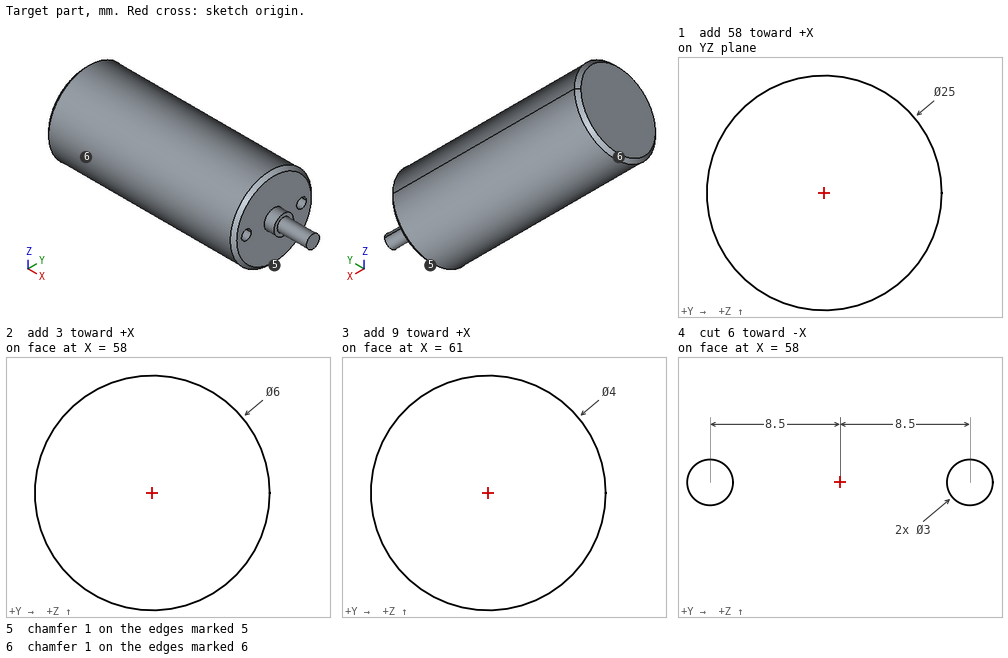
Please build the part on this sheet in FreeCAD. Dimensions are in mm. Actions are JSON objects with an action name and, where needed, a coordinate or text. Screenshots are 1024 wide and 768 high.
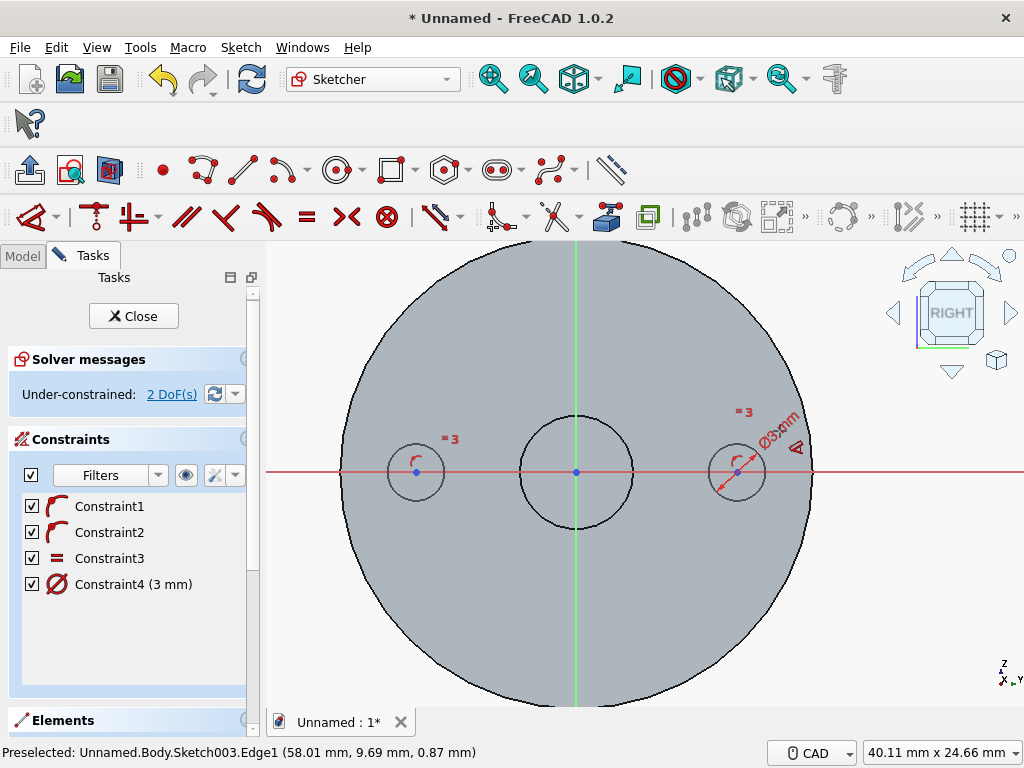
{"action": "left_click", "coordinate": [737, 472]}
{"action": "left_click", "coordinate": [657, 506]}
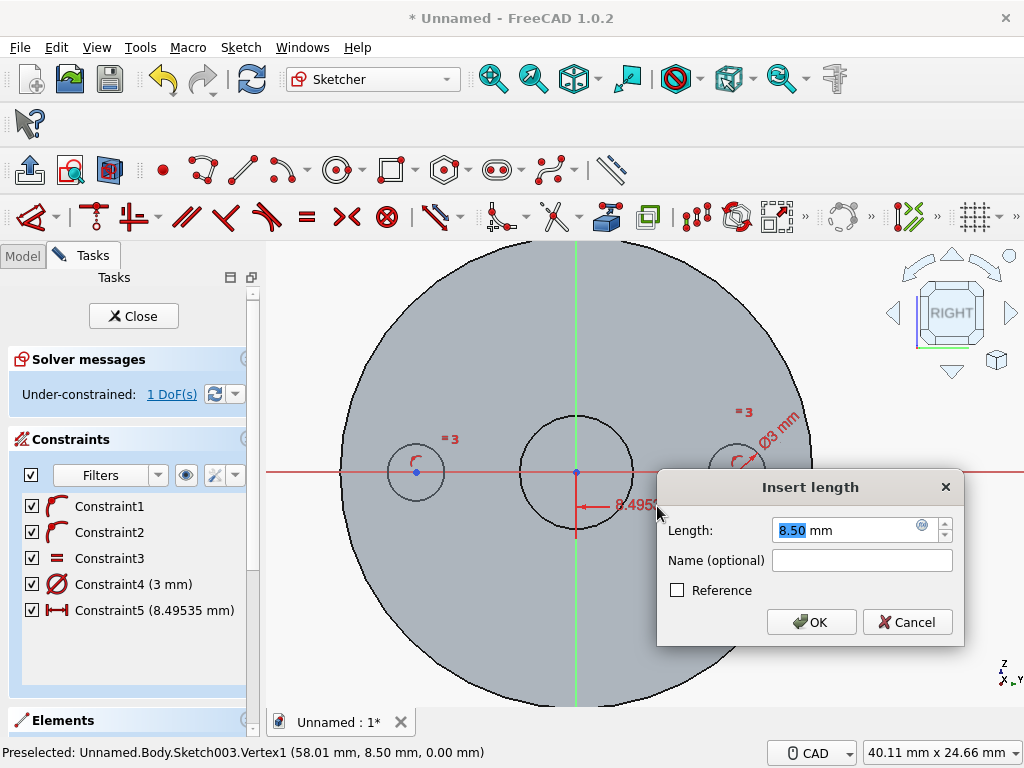
{"action": "type", "text": "8.5"}
{"action": "key", "text": "Return"}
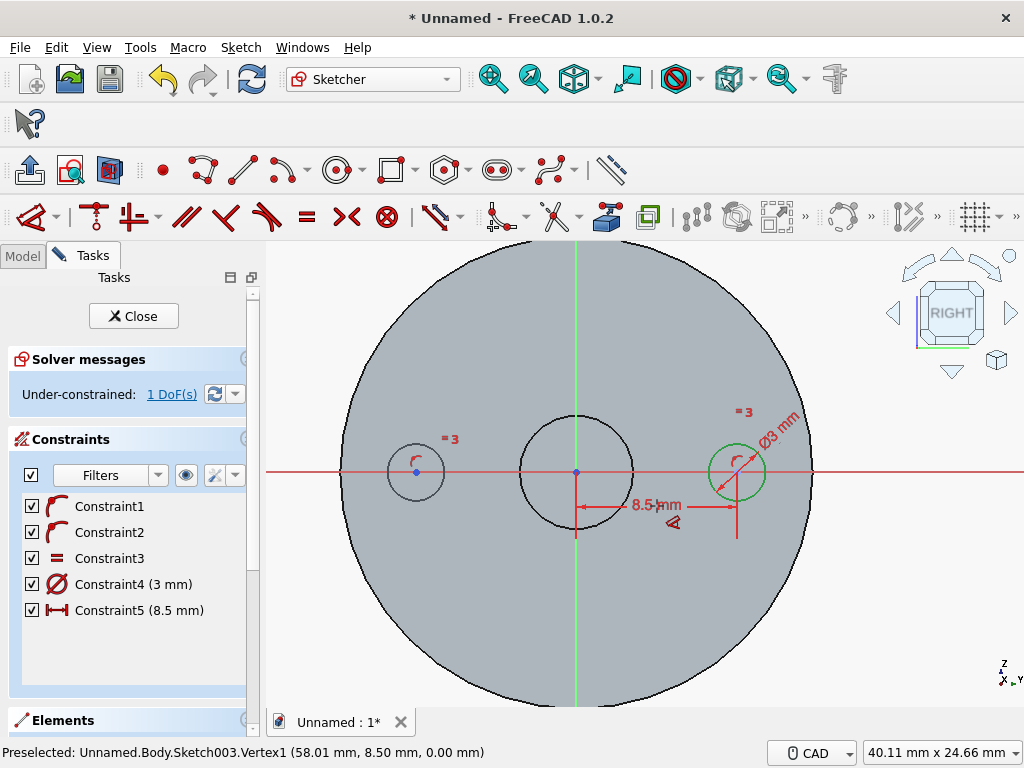
{"action": "left_click", "coordinate": [416, 472]}
{"action": "left_click", "coordinate": [496, 506]}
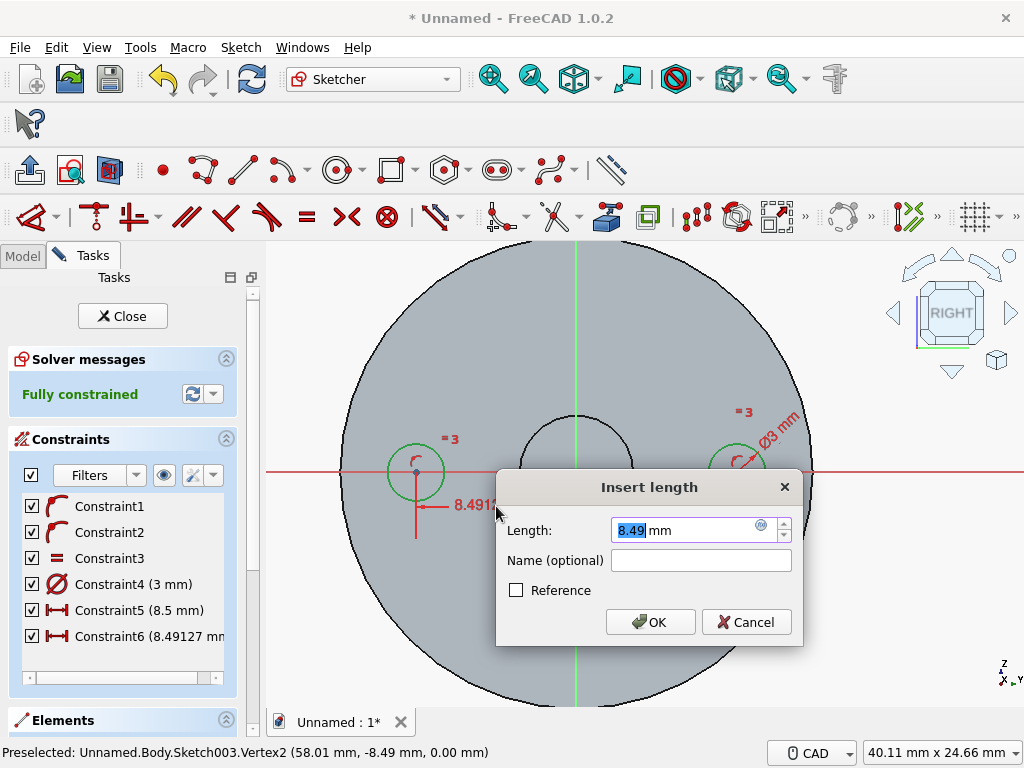
{"action": "type", "text": "8.5"}
{"action": "key", "text": "Return"}
{"action": "key", "text": "Escape"}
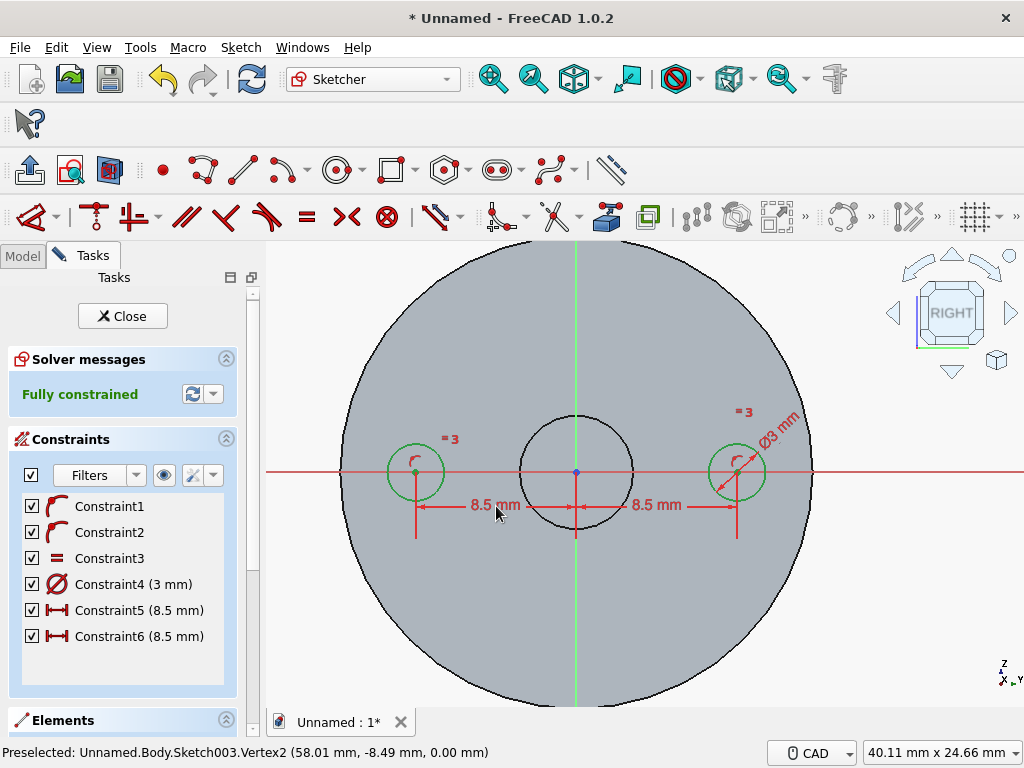
{"action": "left_click", "coordinate": [123, 316]}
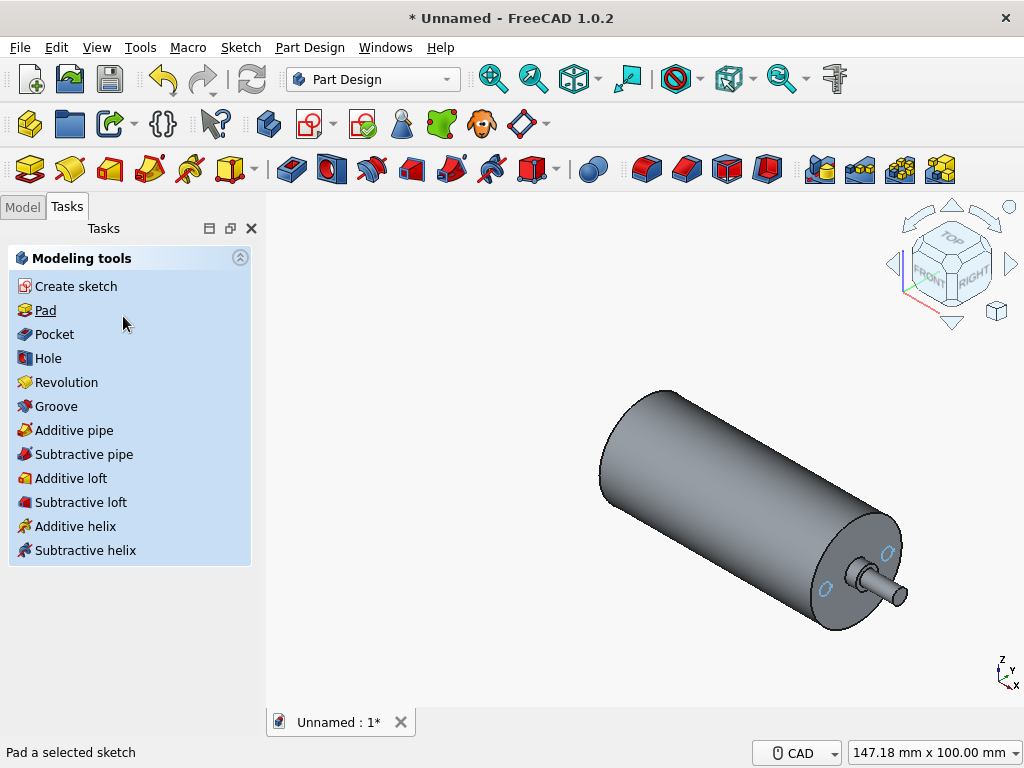
{"action": "left_click", "coordinate": [292, 170]}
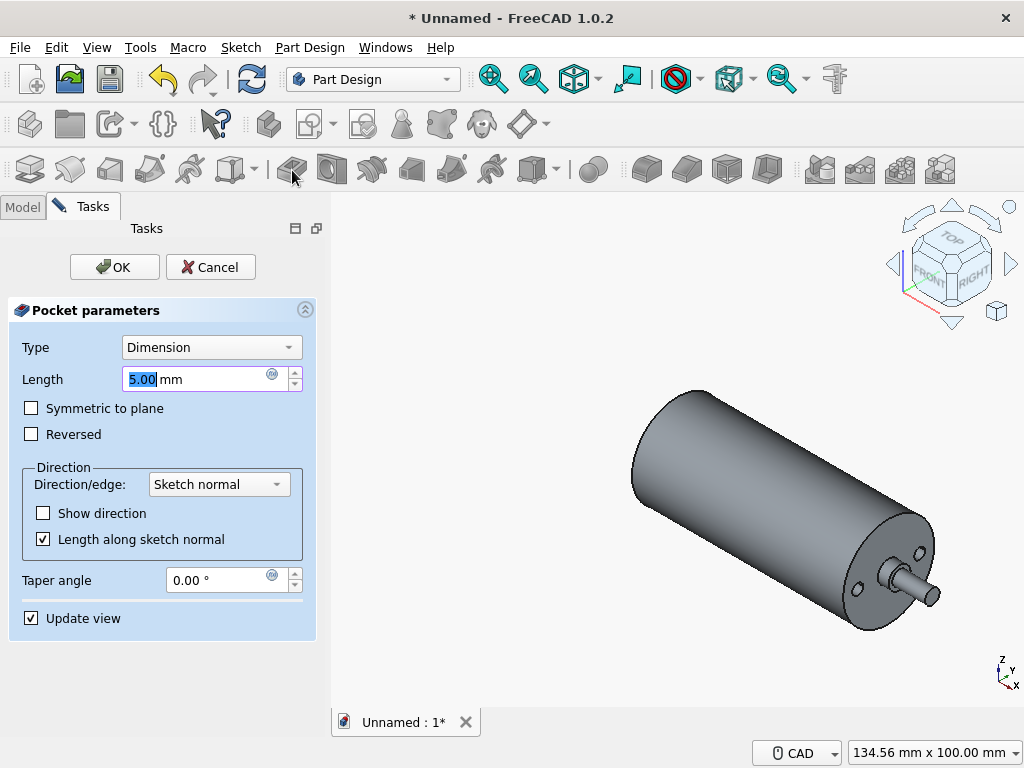
{"action": "type", "text": "6"}
{"action": "key", "text": "Tab"}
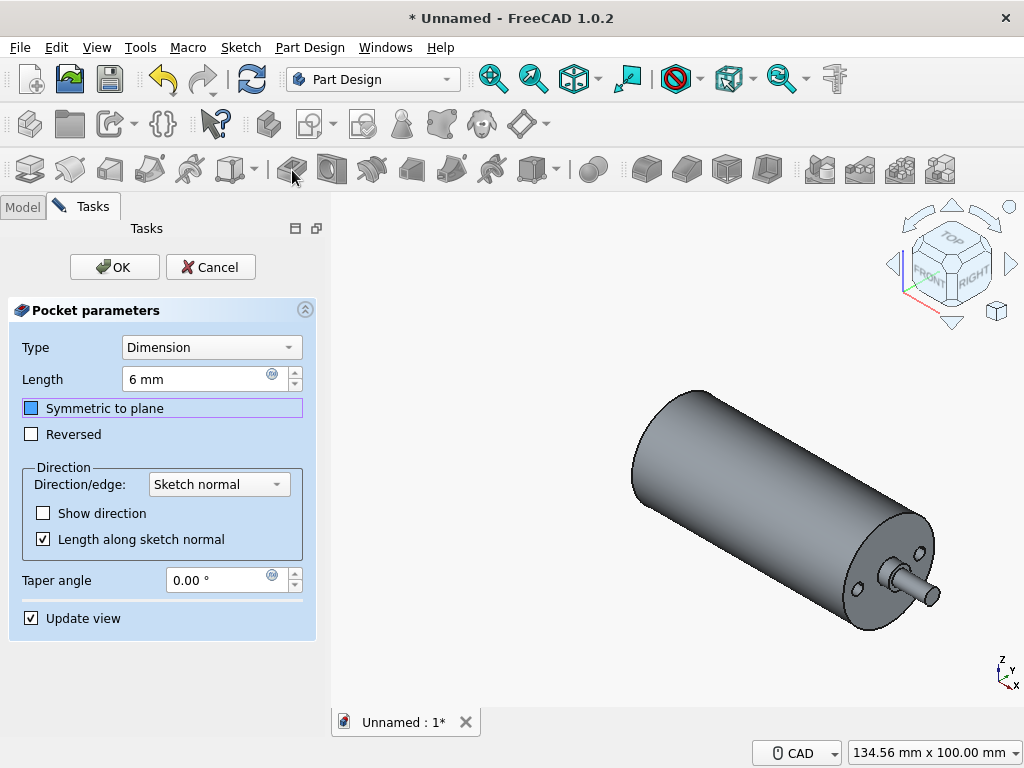
{"action": "left_click", "coordinate": [115, 267]}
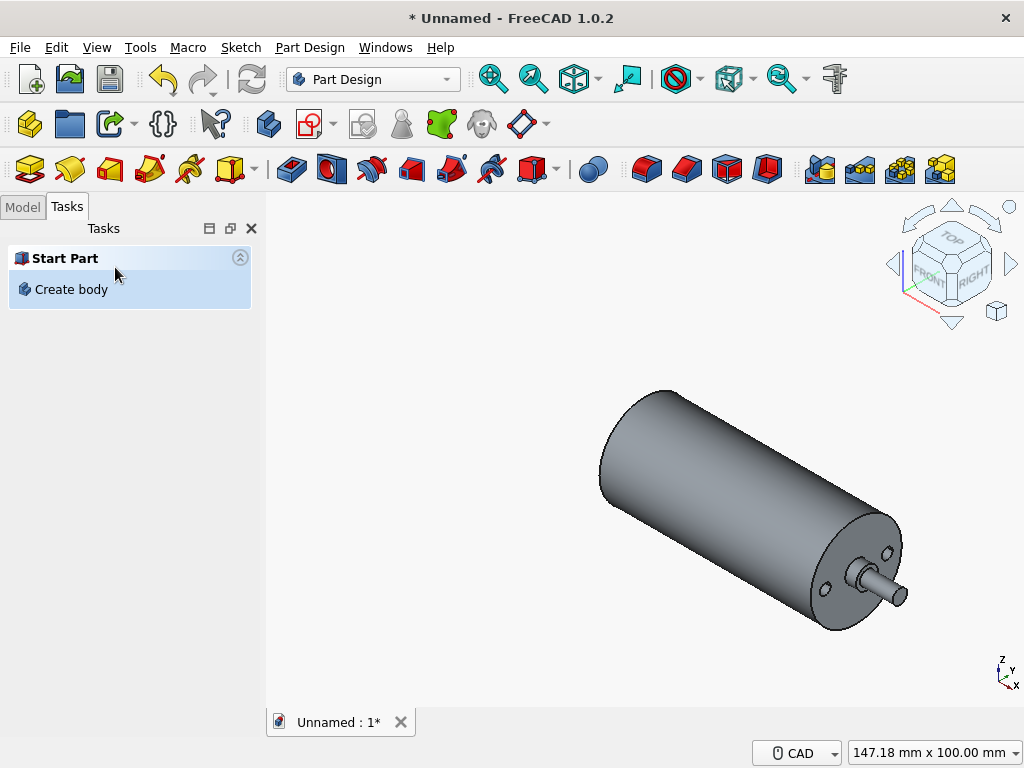
{"action": "left_click", "coordinate": [811, 597]}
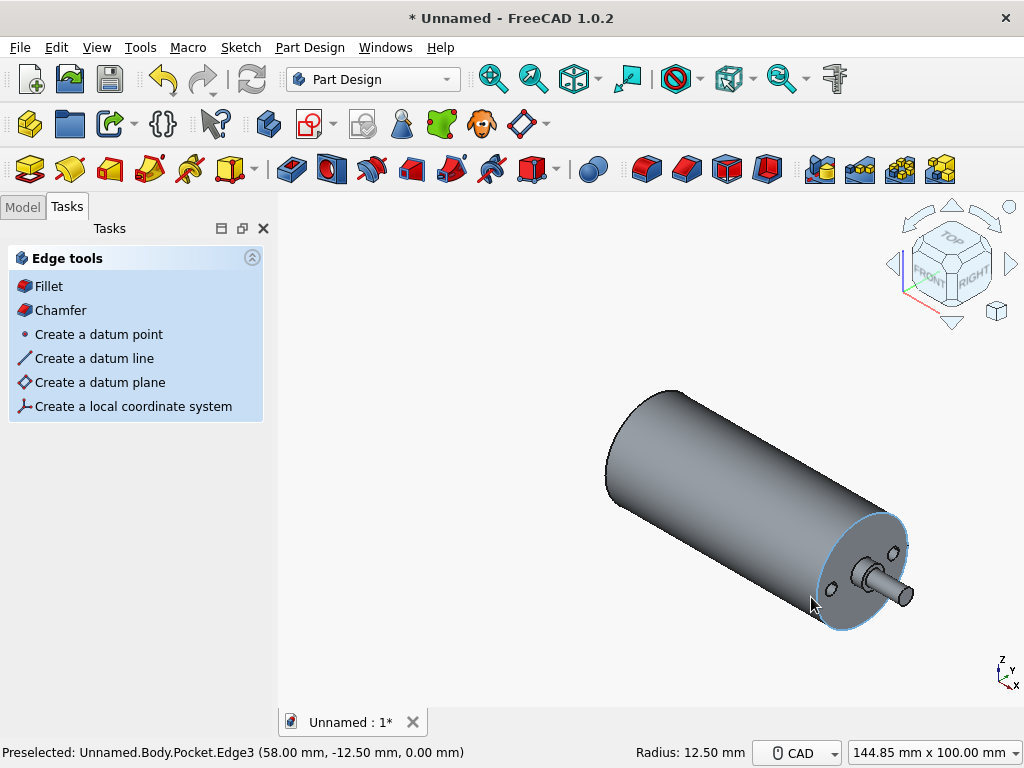
{"action": "left_click", "coordinate": [688, 170]}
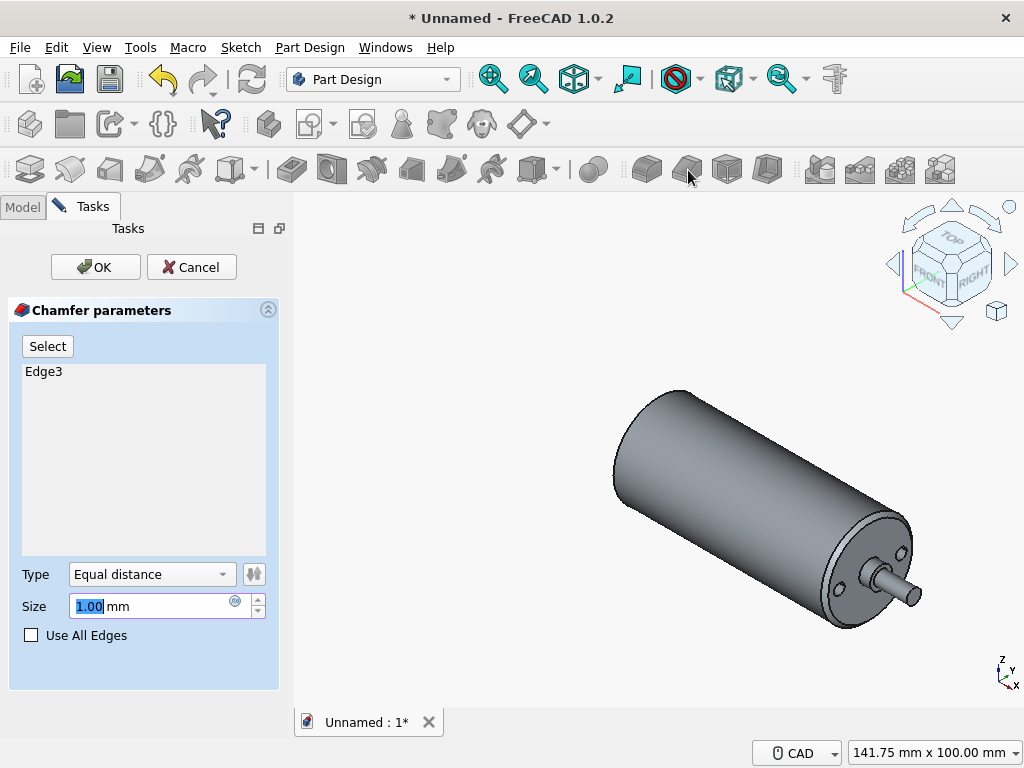
{"action": "type", "text": "1"}
{"action": "key", "text": "Tab"}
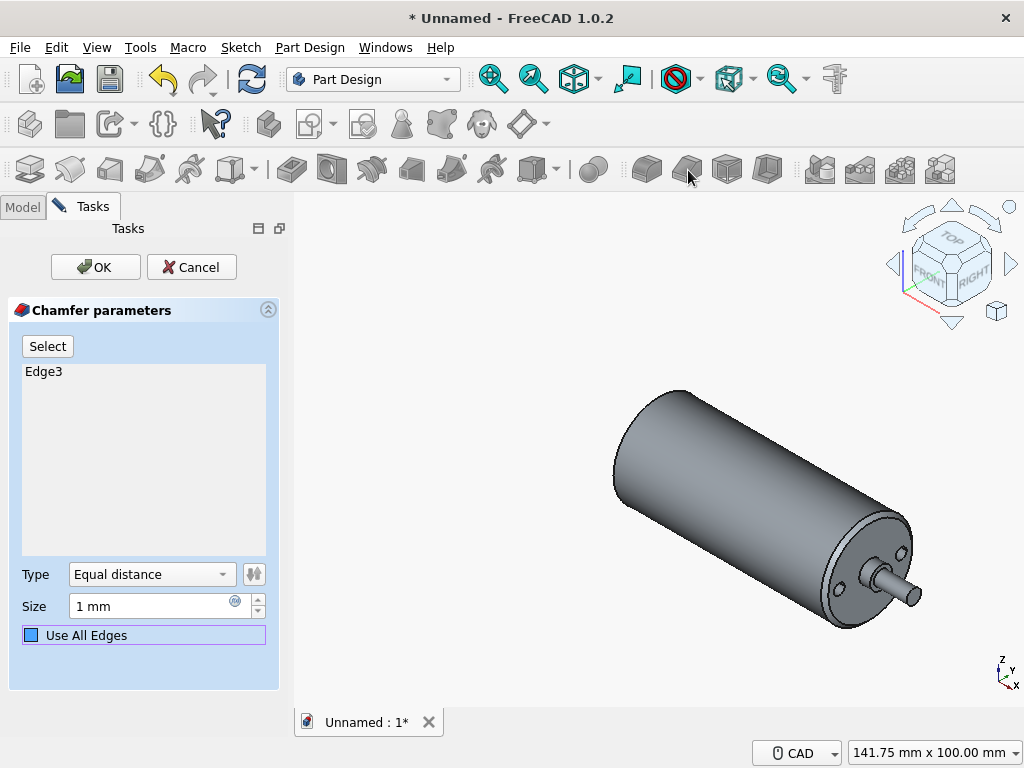
{"action": "left_click", "coordinate": [96, 267]}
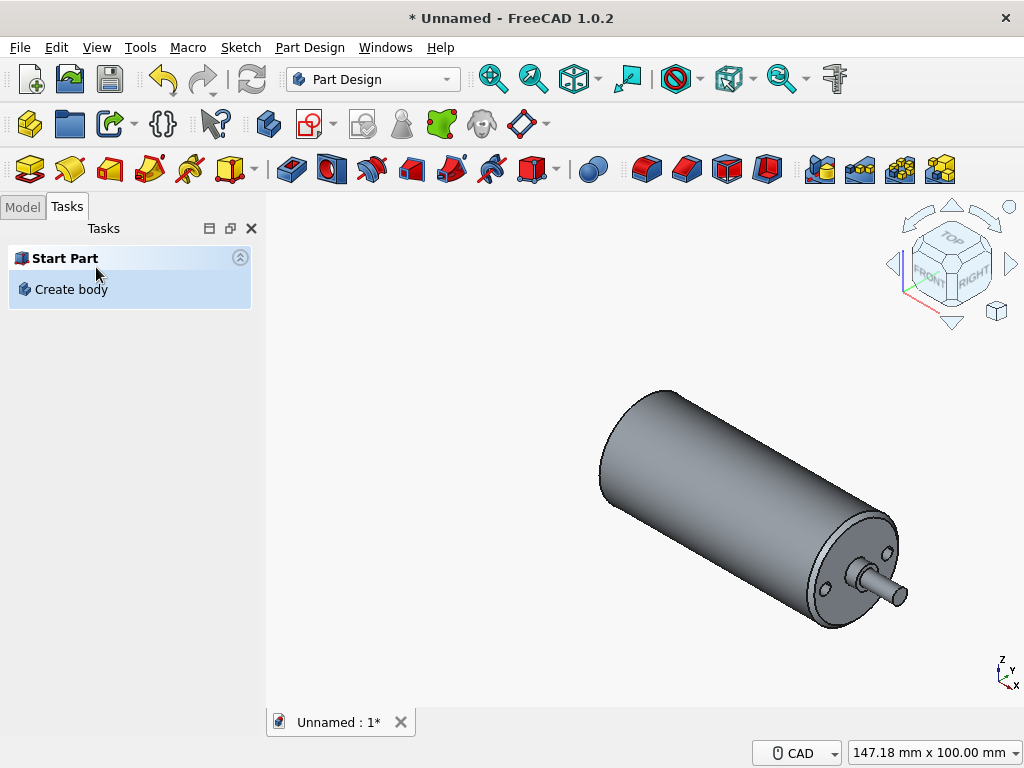
{"action": "key", "text": "2"}